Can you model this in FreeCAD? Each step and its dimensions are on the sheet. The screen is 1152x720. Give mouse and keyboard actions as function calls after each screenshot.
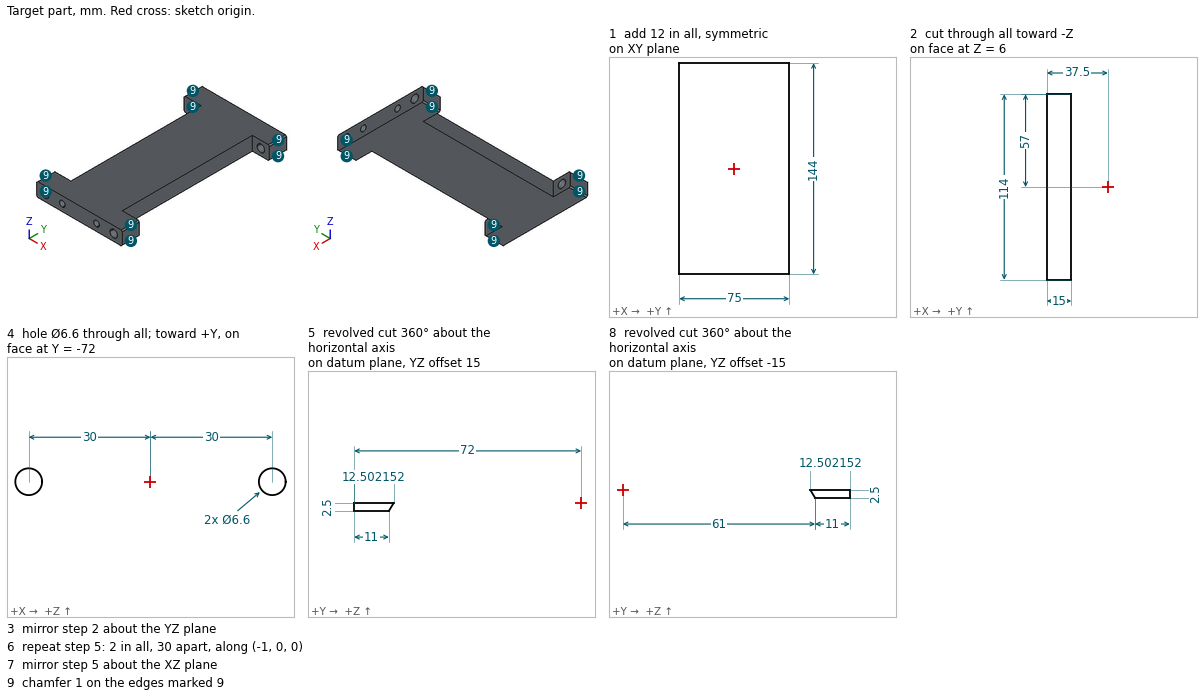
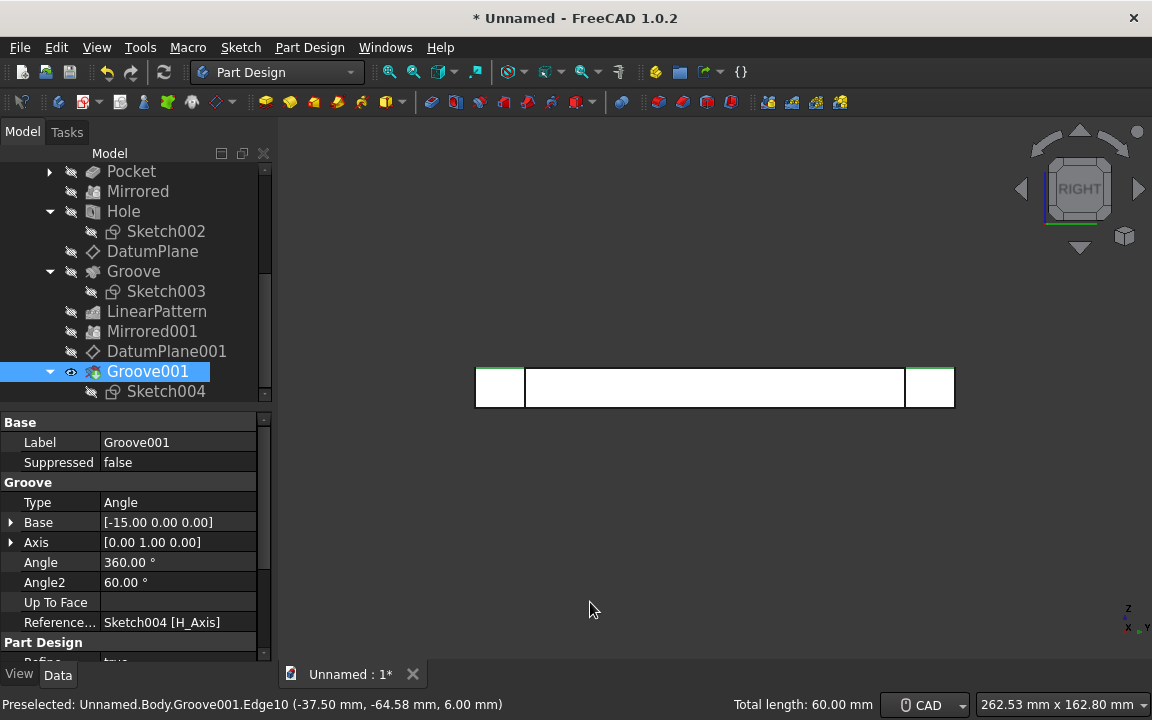
click(930, 407, ctrl)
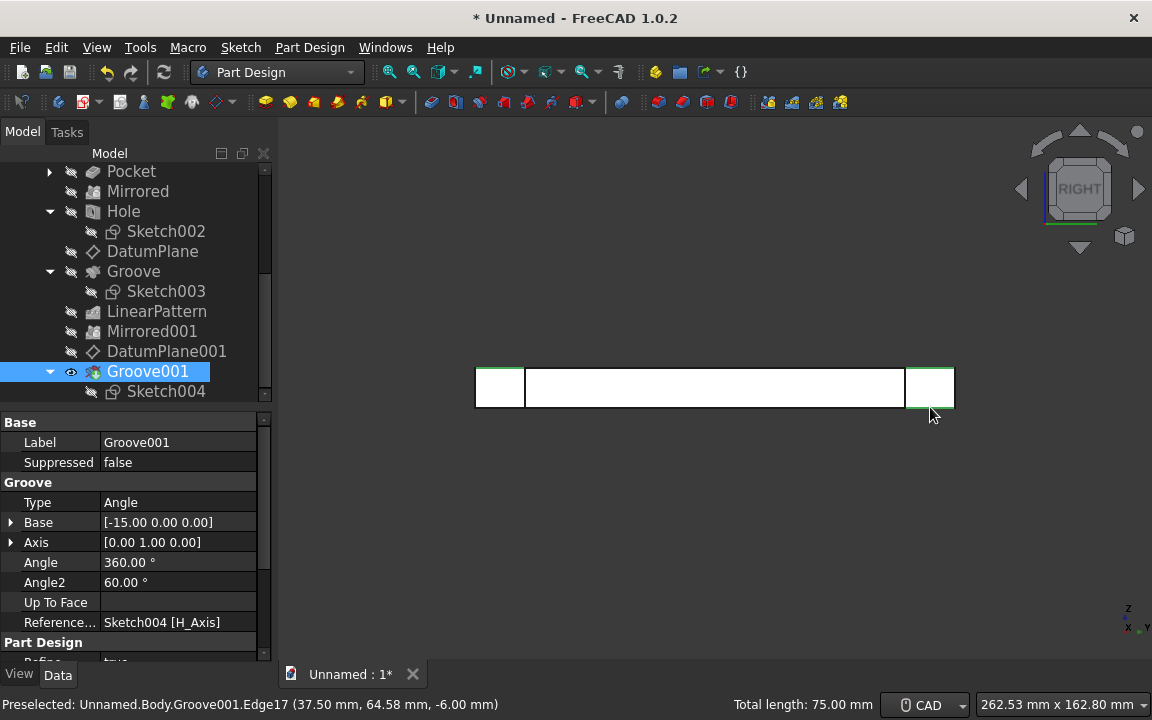
click(500, 407, ctrl)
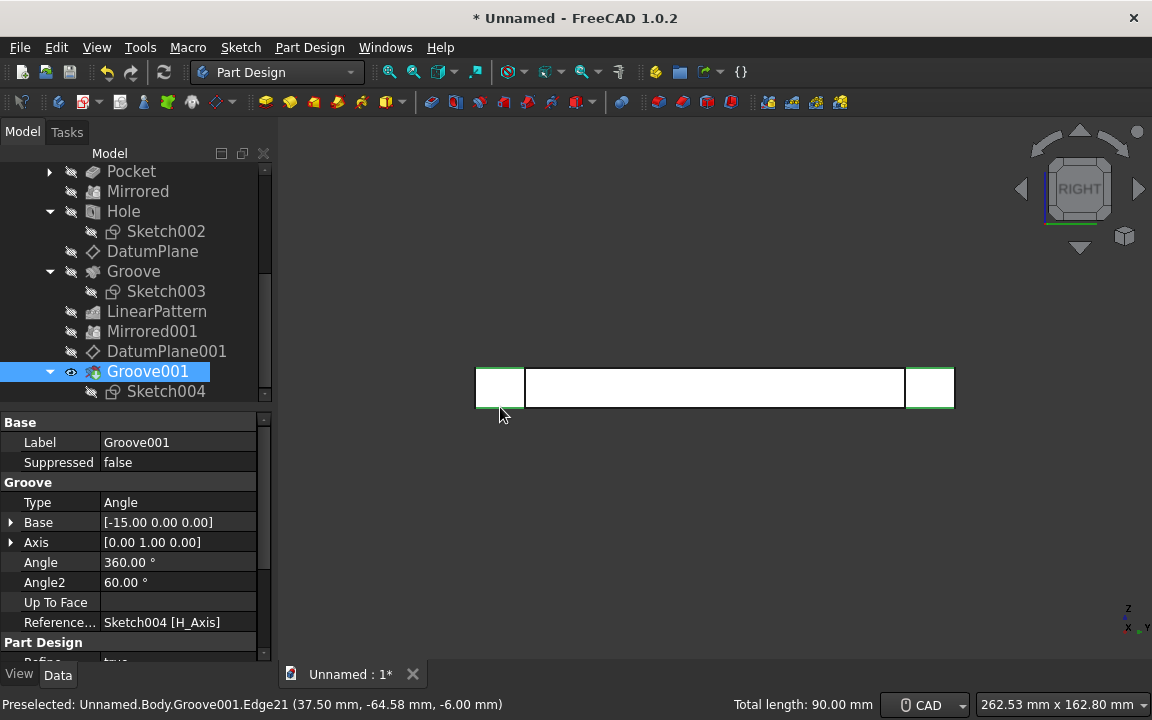
key(5)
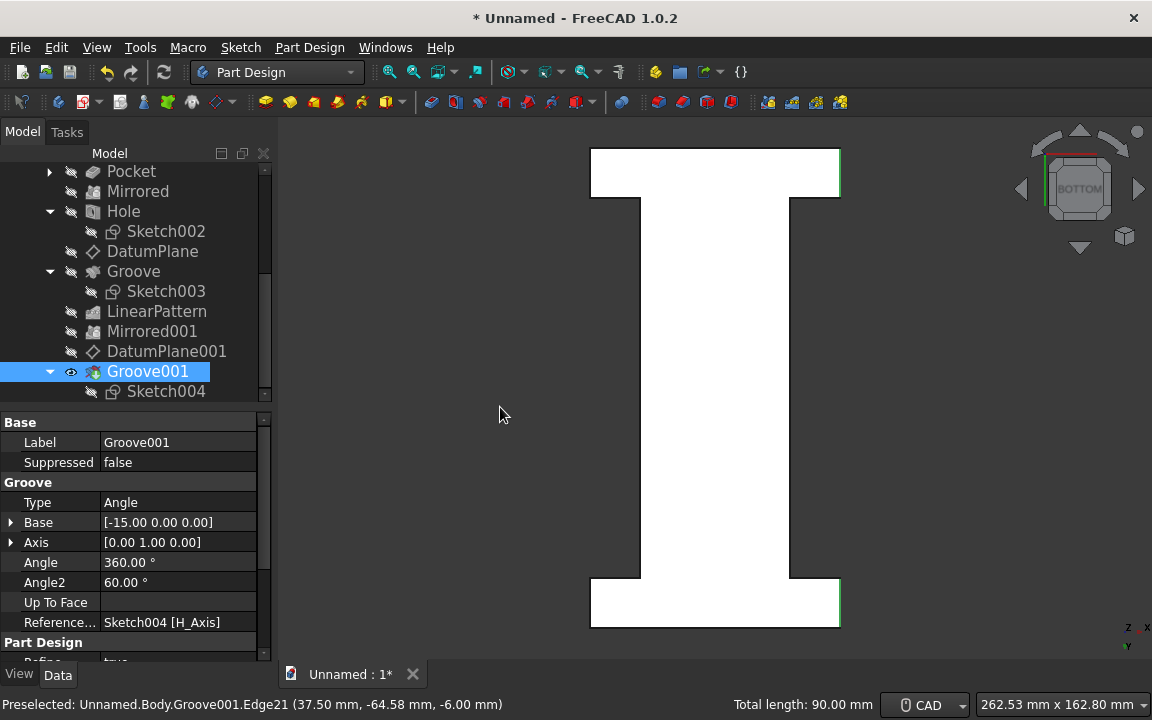
click(590, 172, ctrl)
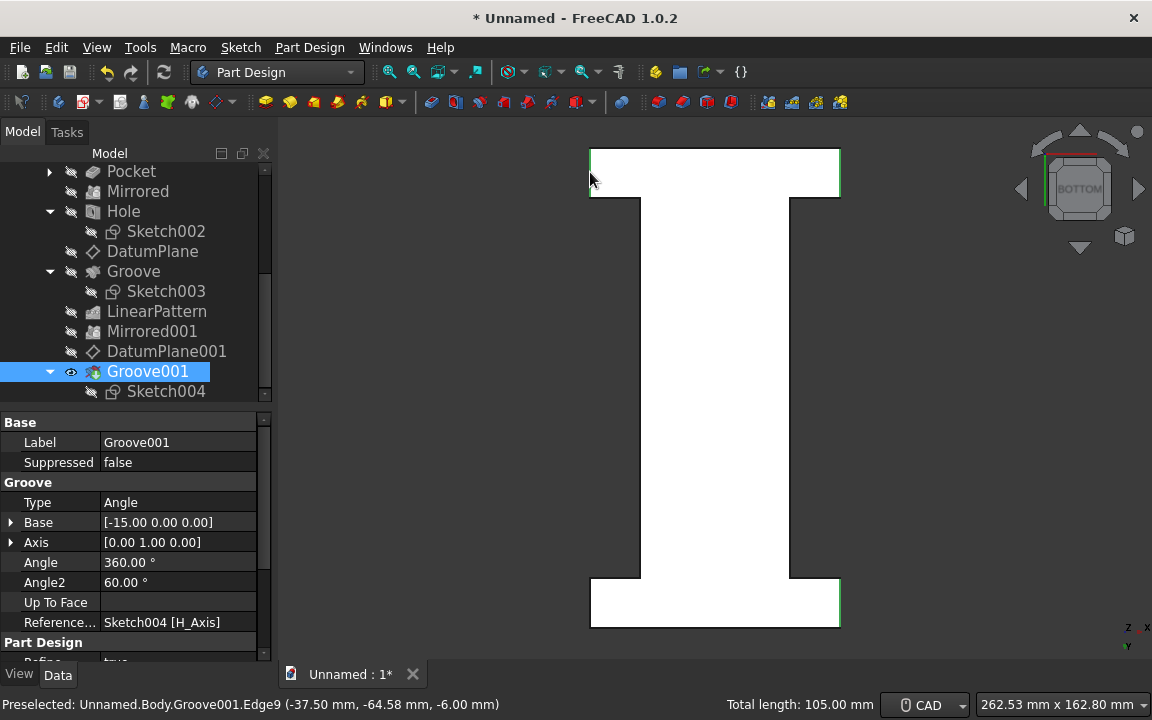
click(590, 602, ctrl)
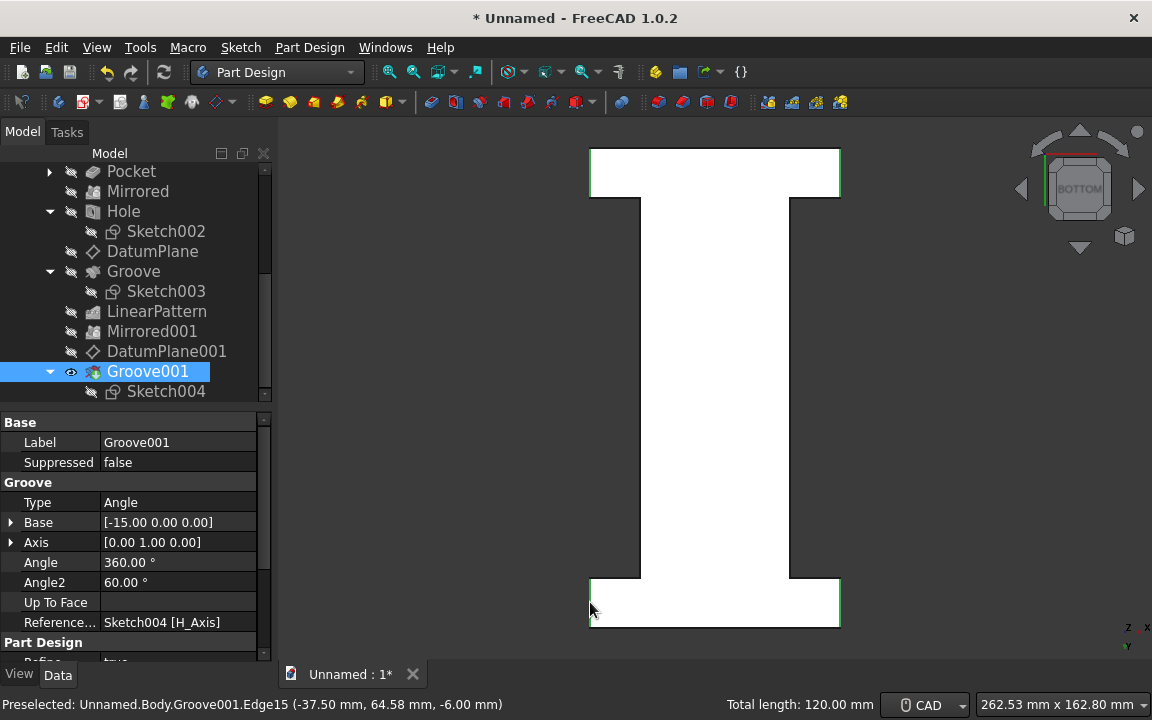
click(684, 102)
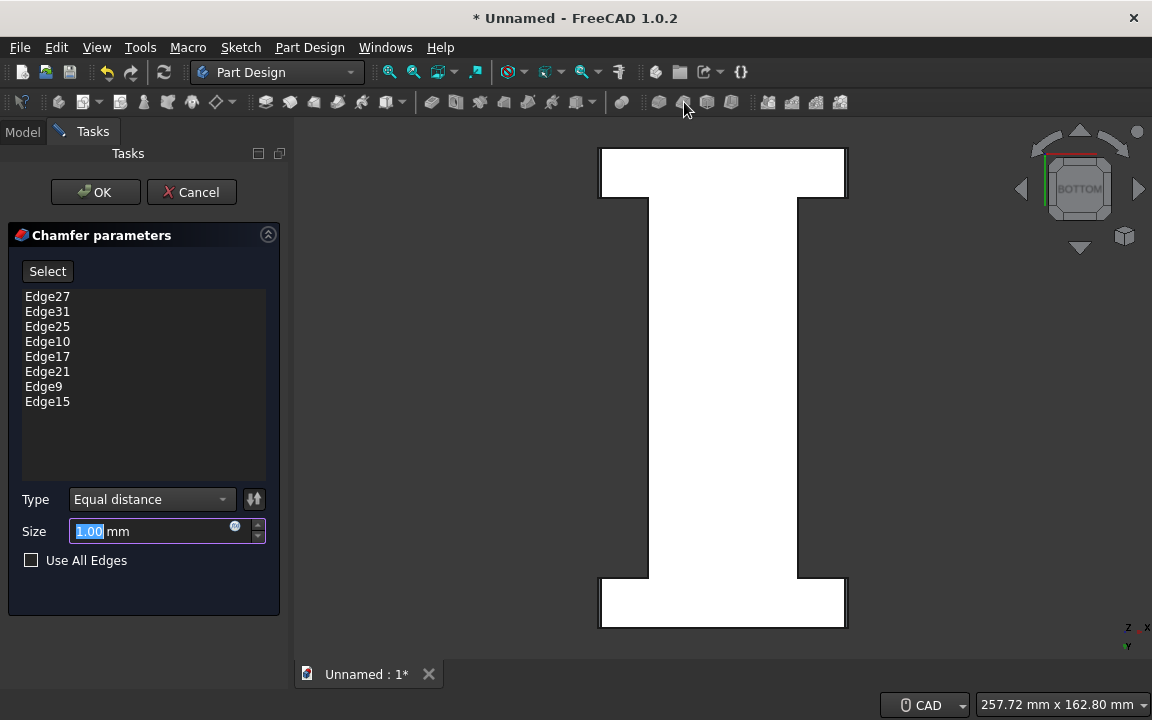
text(1)
key(Tab)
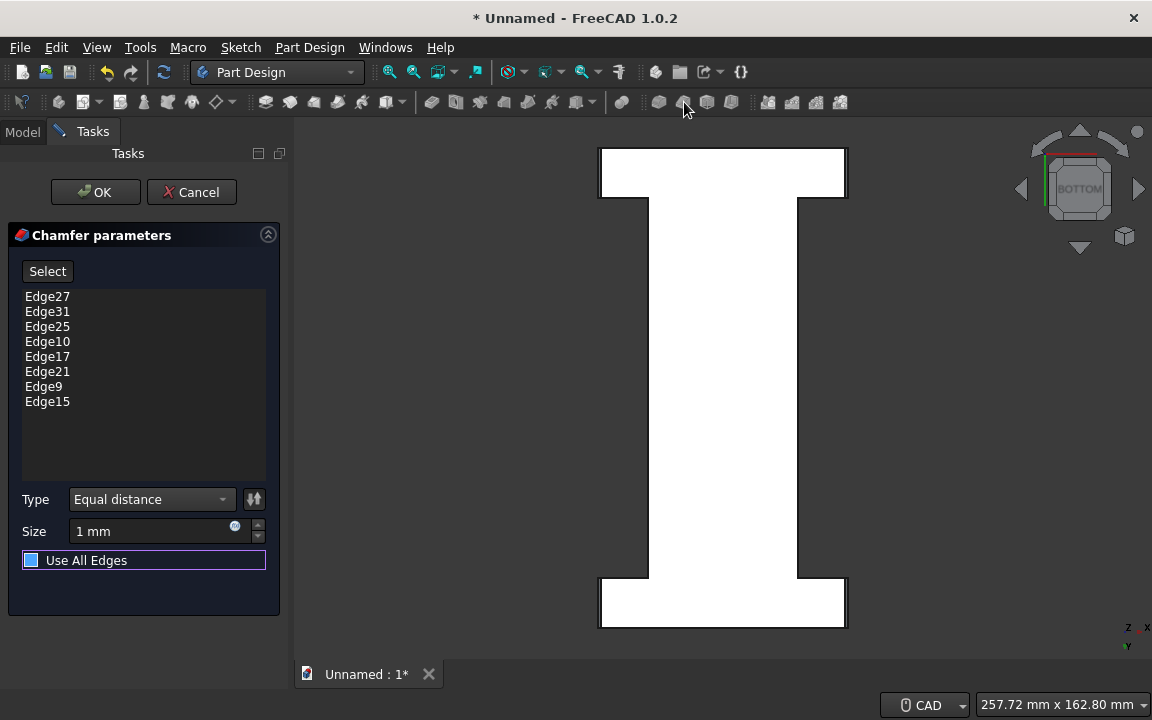
click(96, 192)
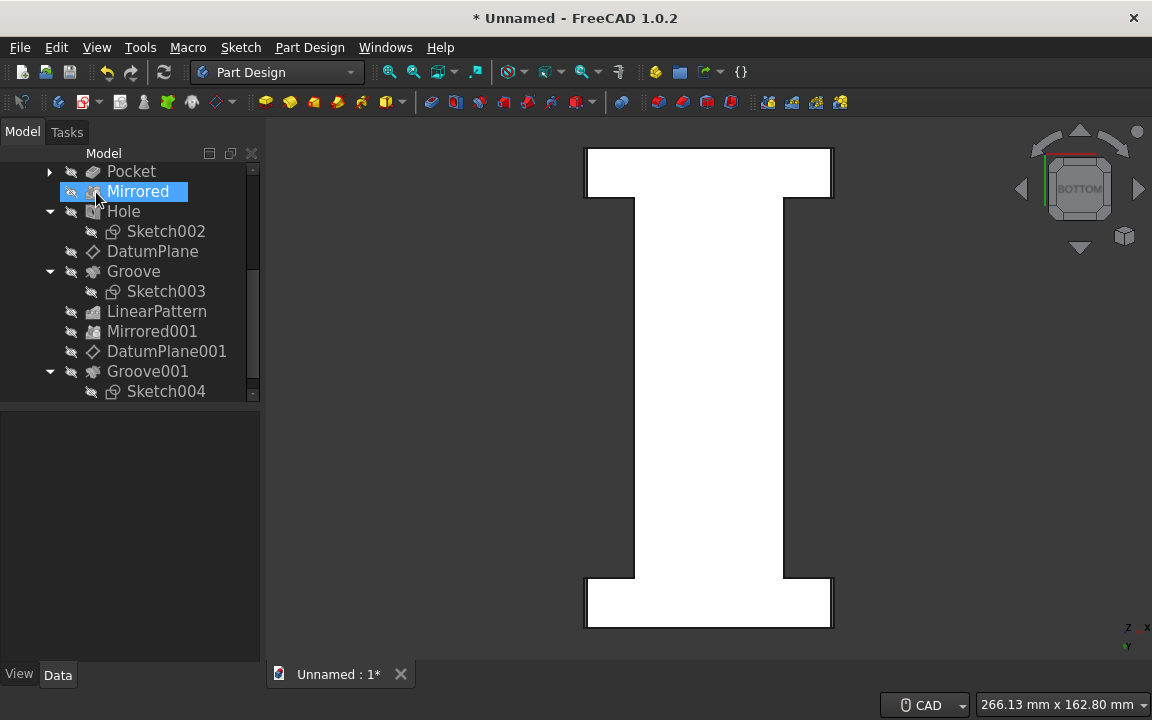
key(0)